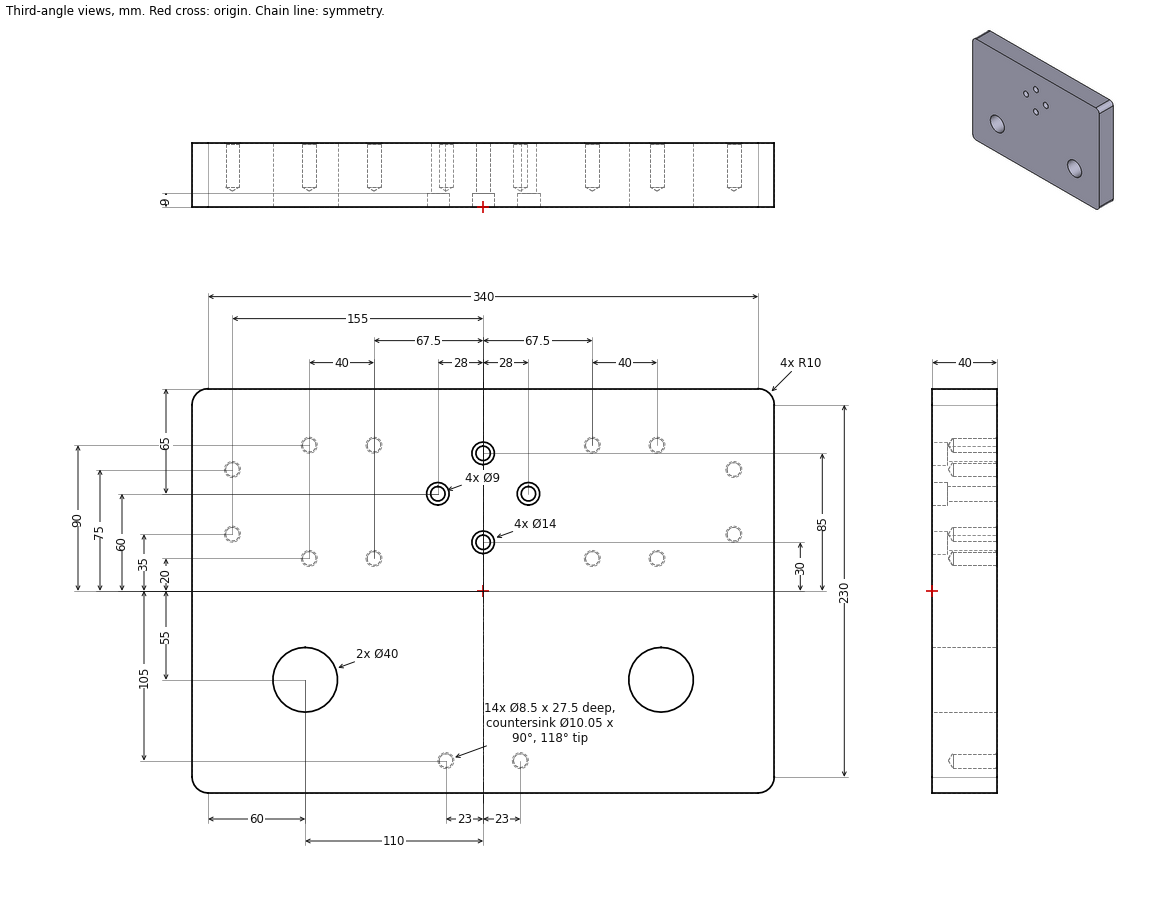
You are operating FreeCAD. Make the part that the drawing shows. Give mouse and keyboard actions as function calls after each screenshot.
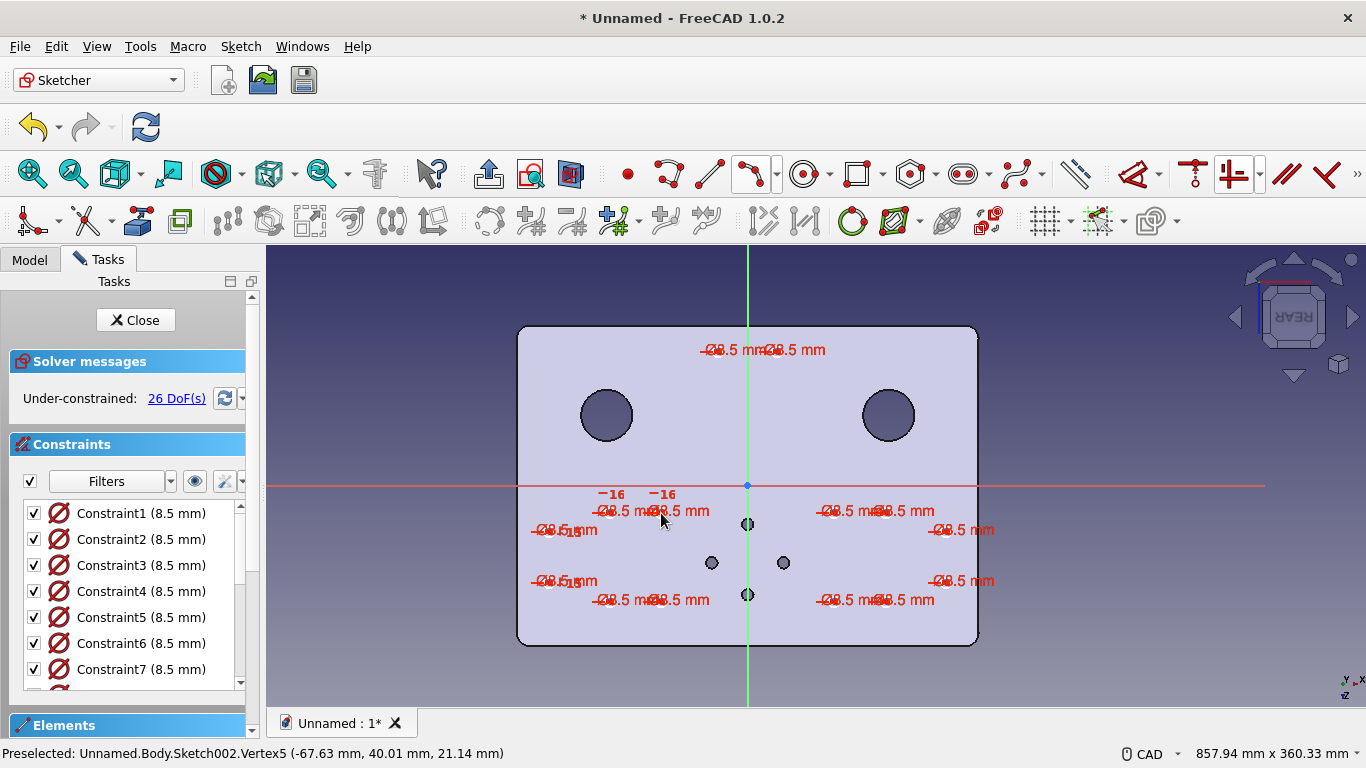
click(610, 513)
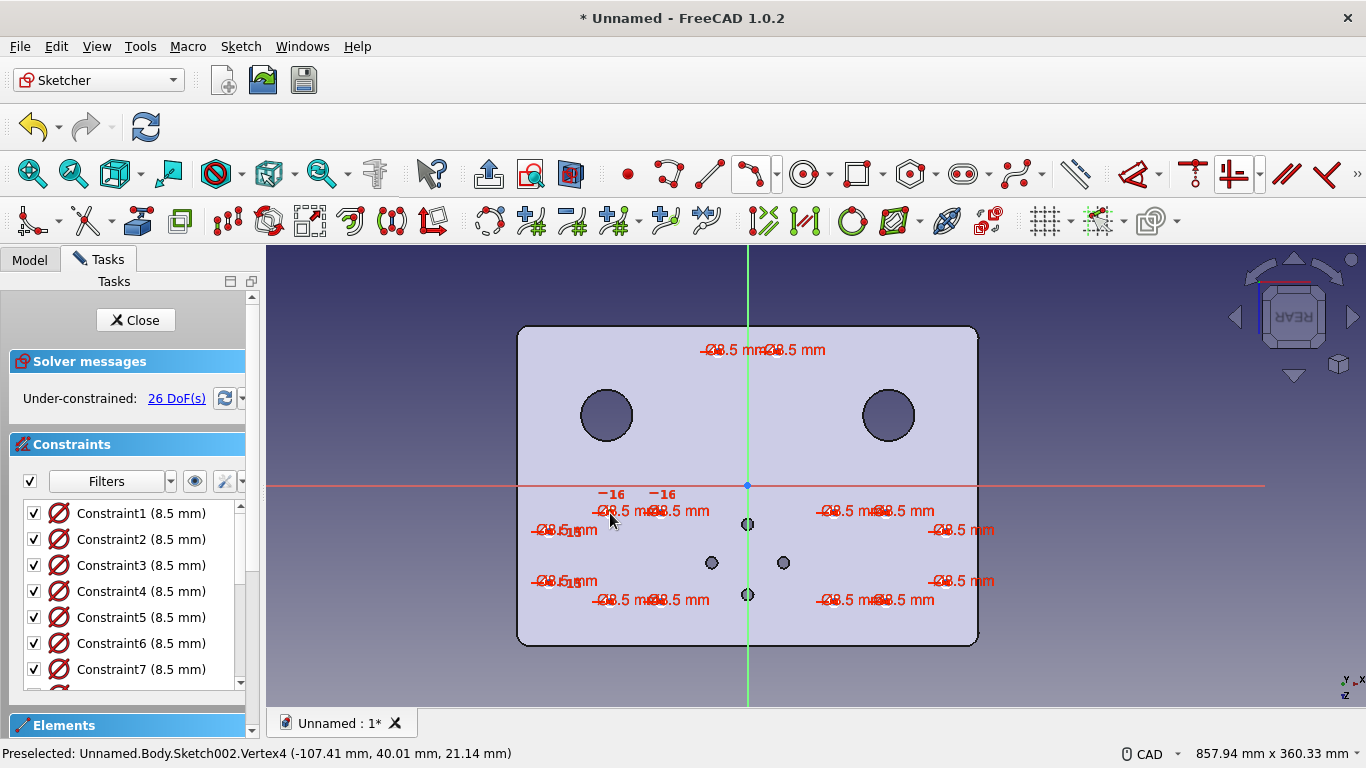
click(610, 602)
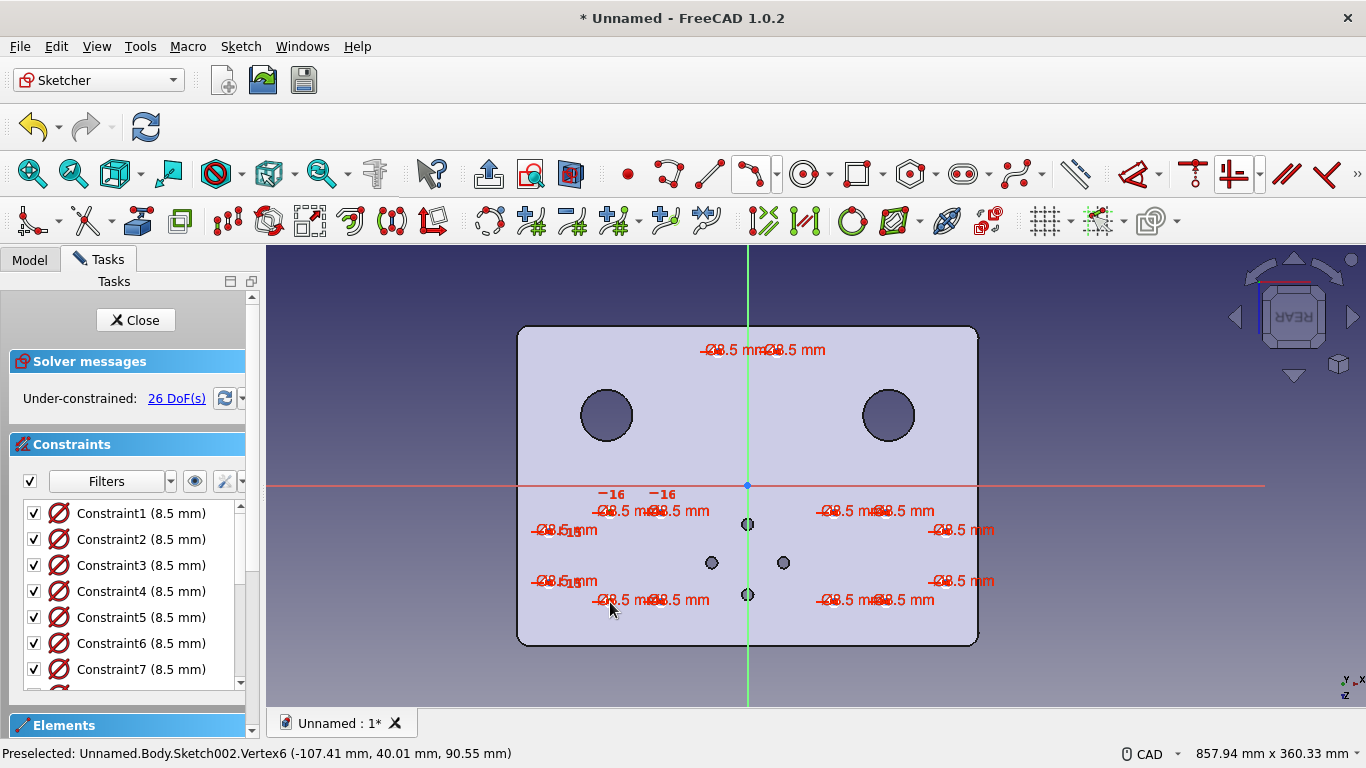
click(1260, 174)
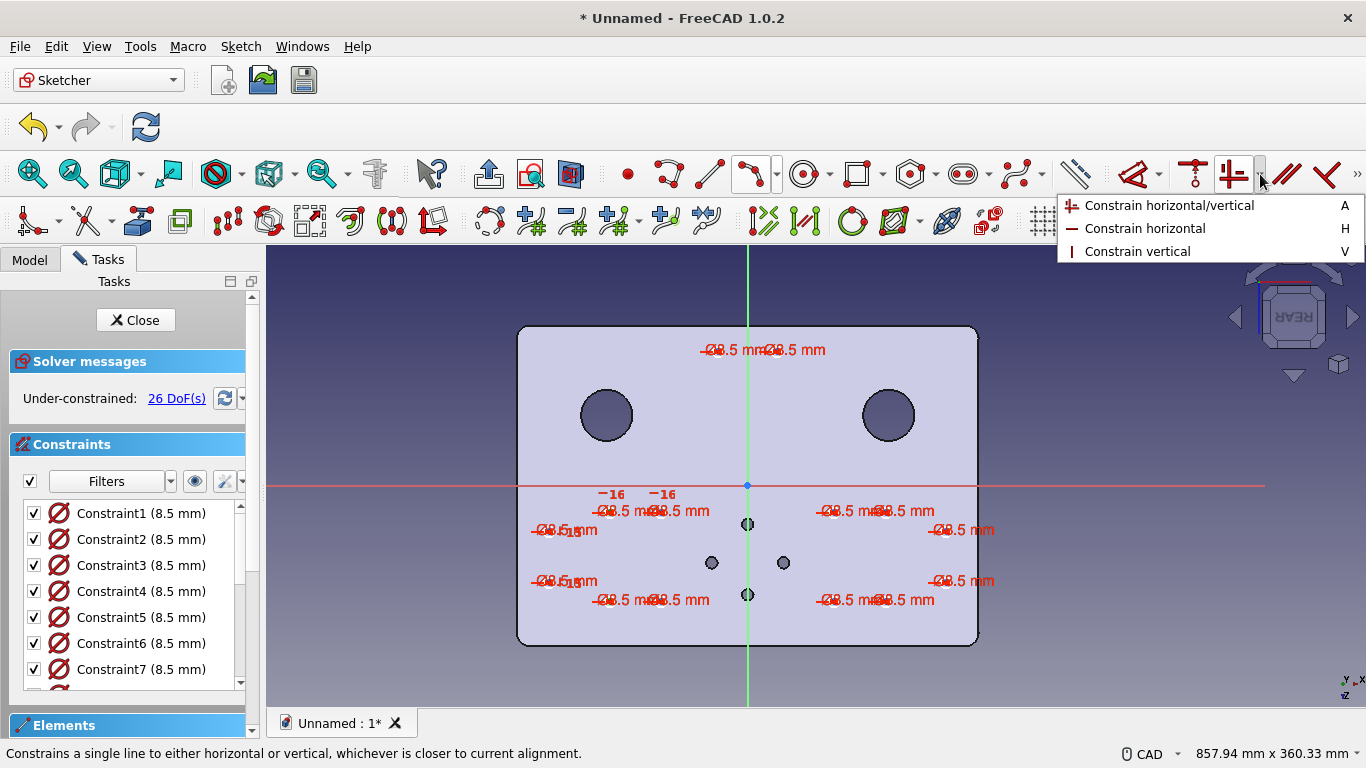
click(1211, 252)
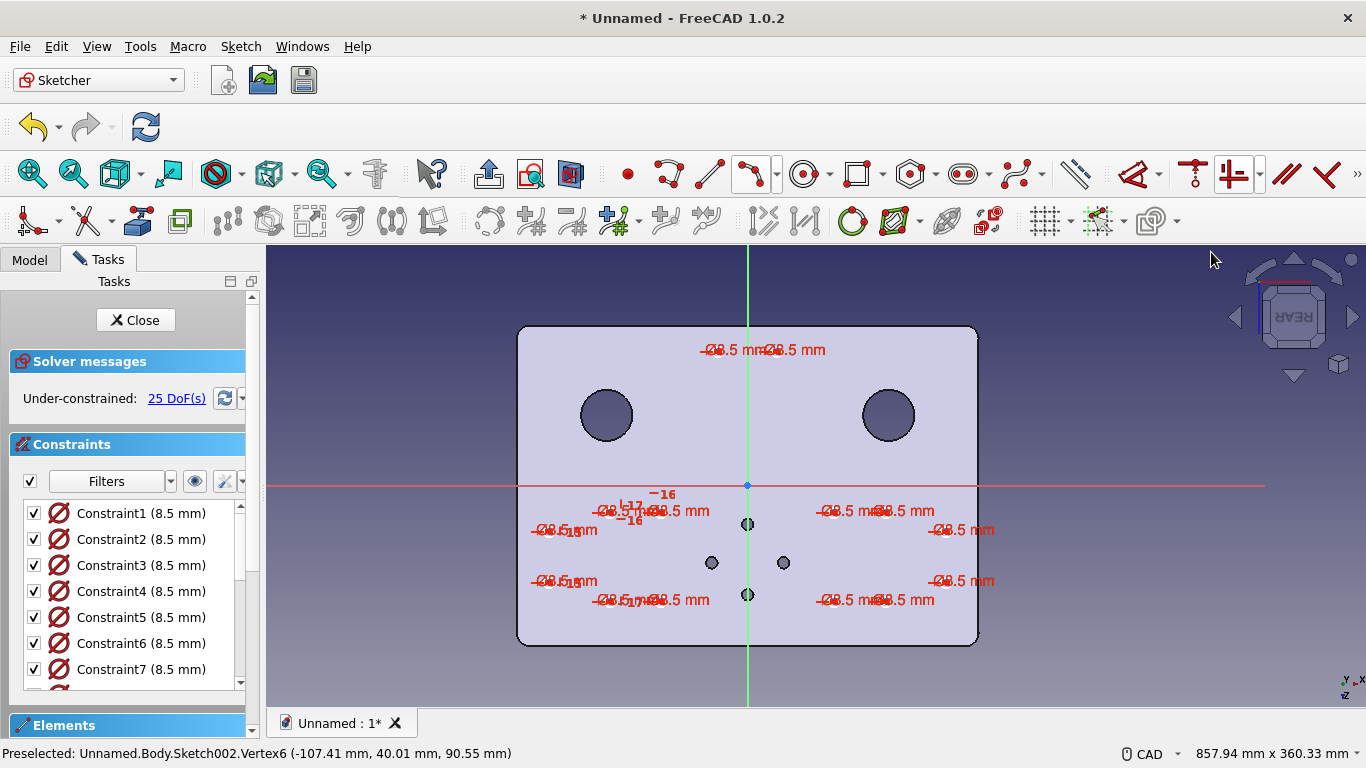
click(661, 513)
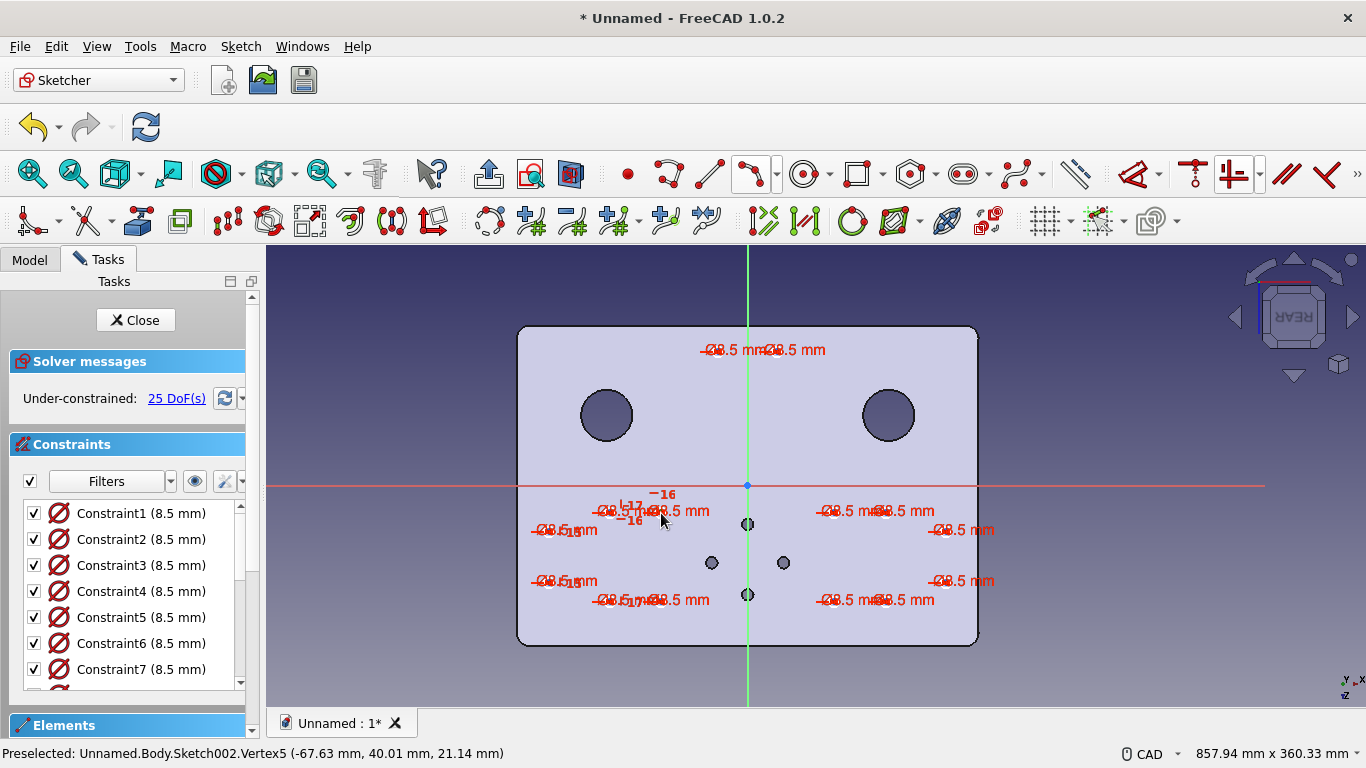
click(661, 602)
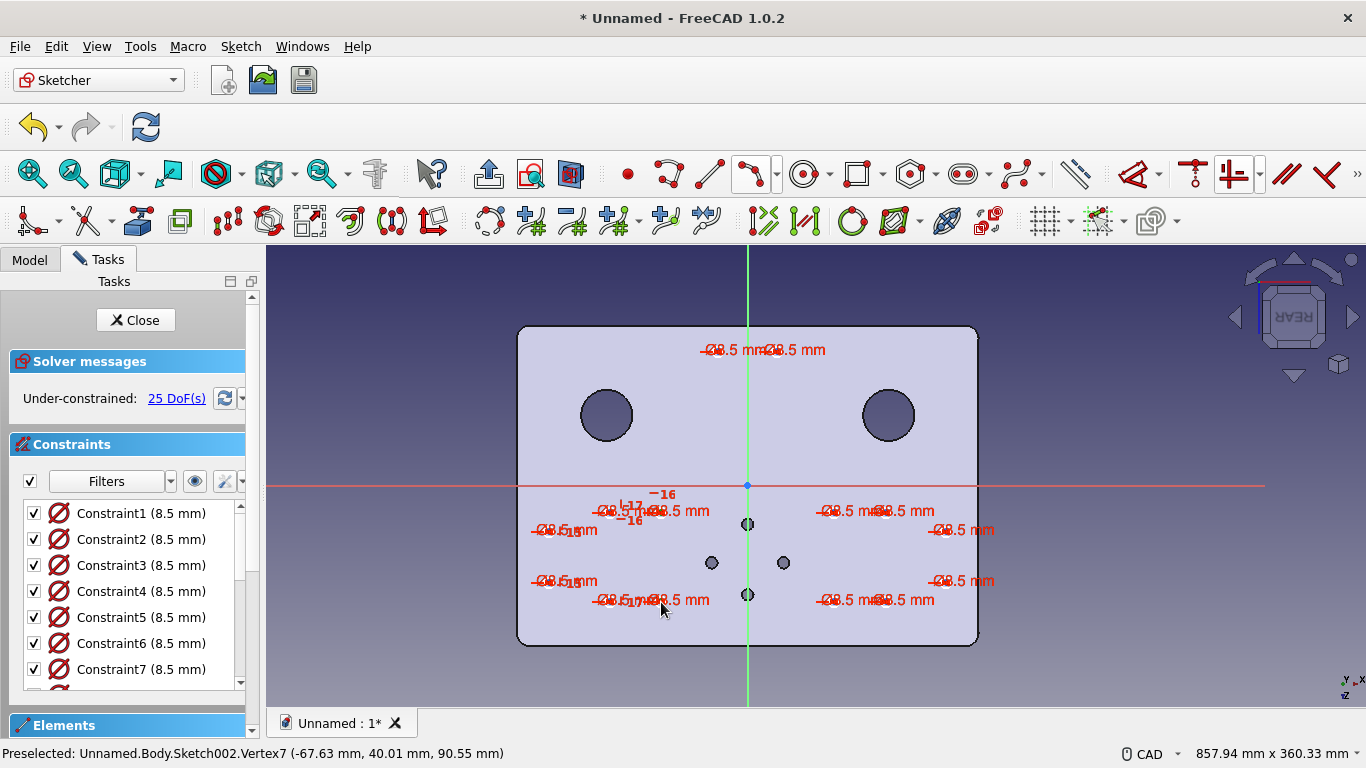
key(v)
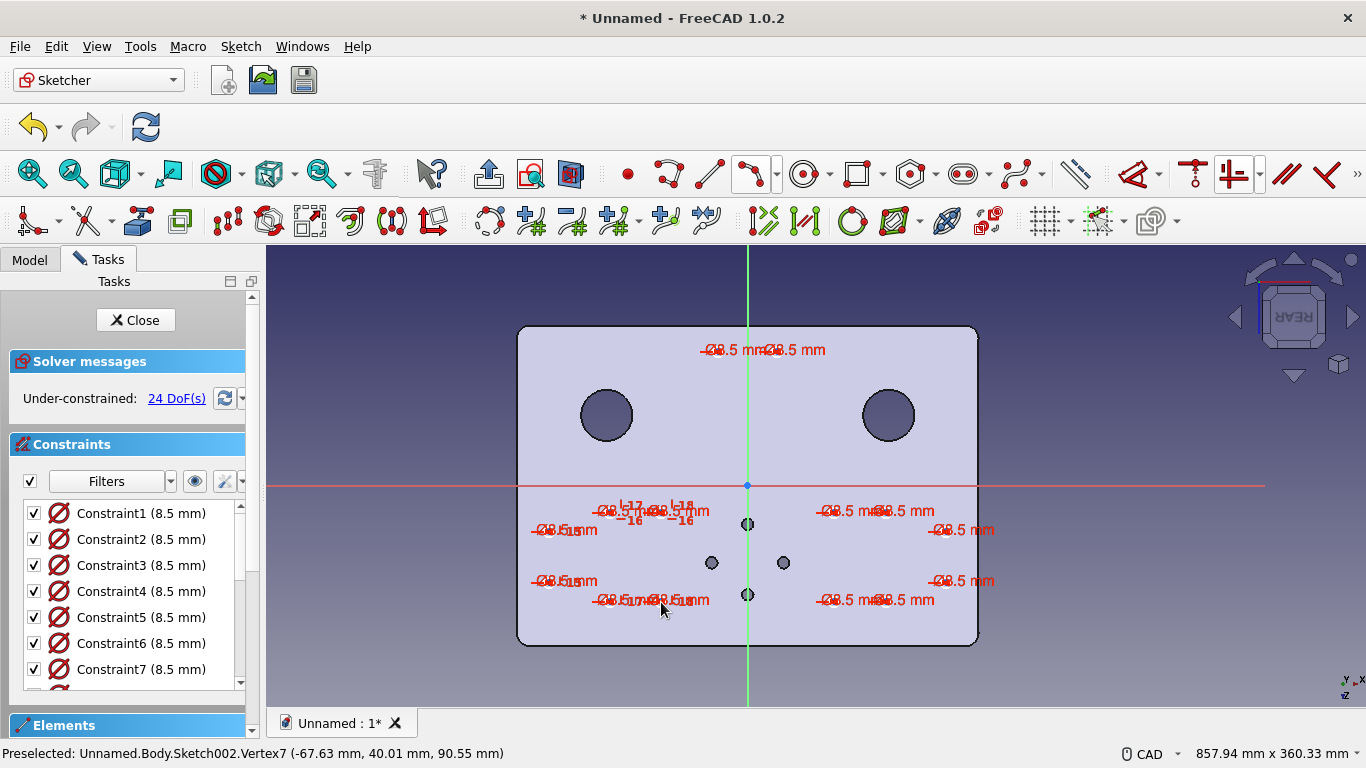
click(610, 602)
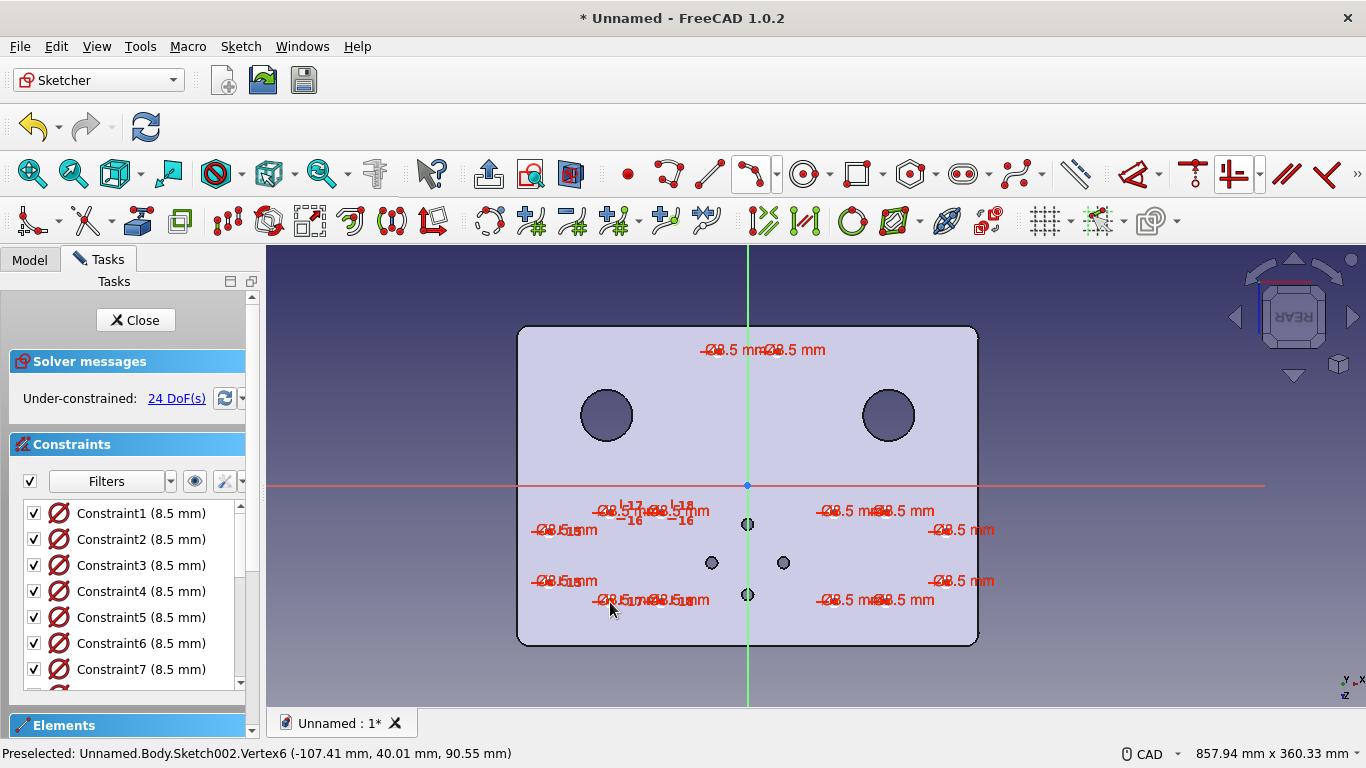
click(661, 602)